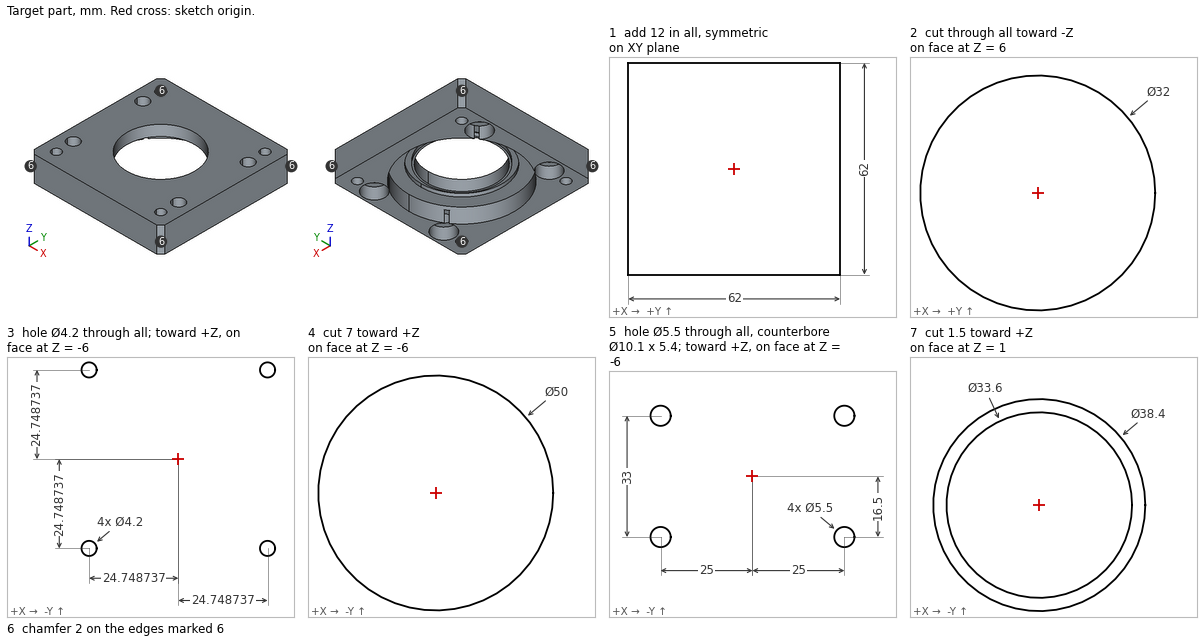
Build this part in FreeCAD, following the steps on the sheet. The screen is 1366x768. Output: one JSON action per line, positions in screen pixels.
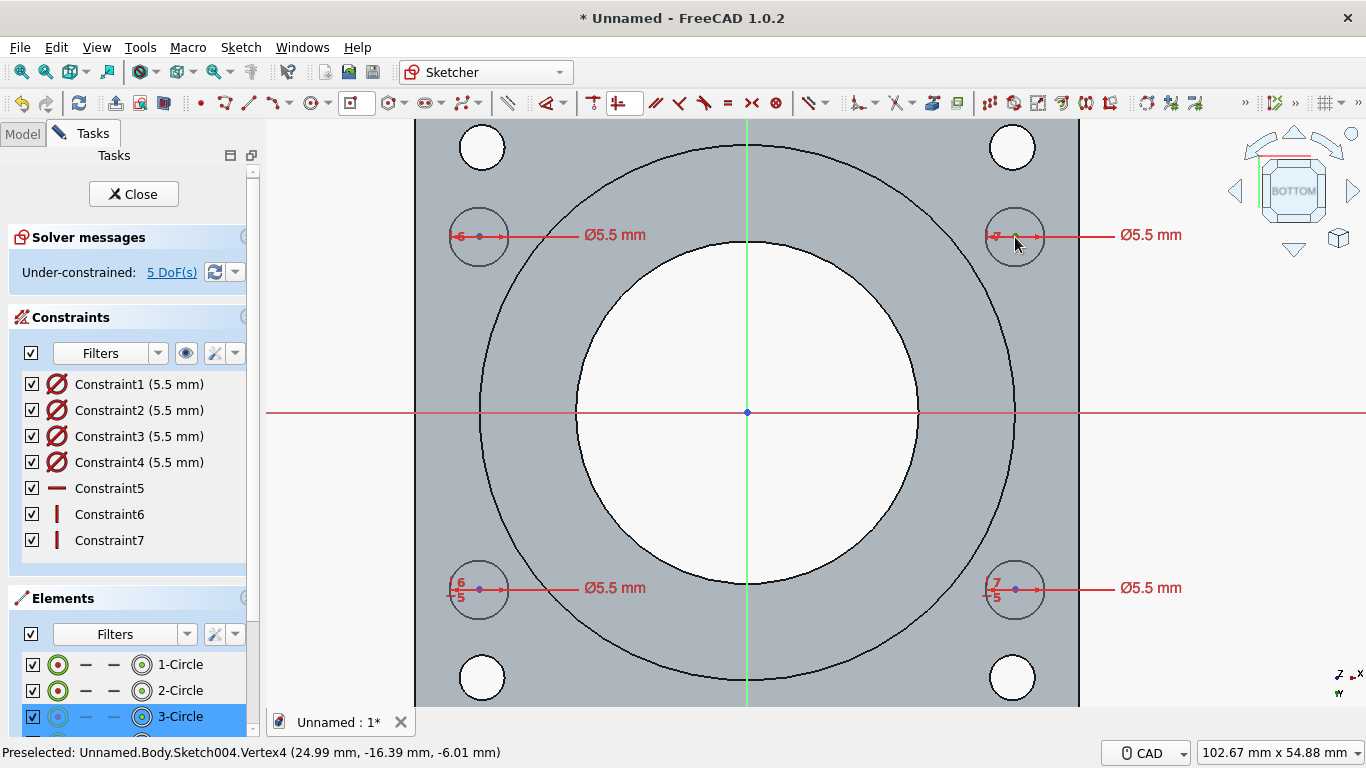
{"action": "left_click", "coordinate": [638, 104]}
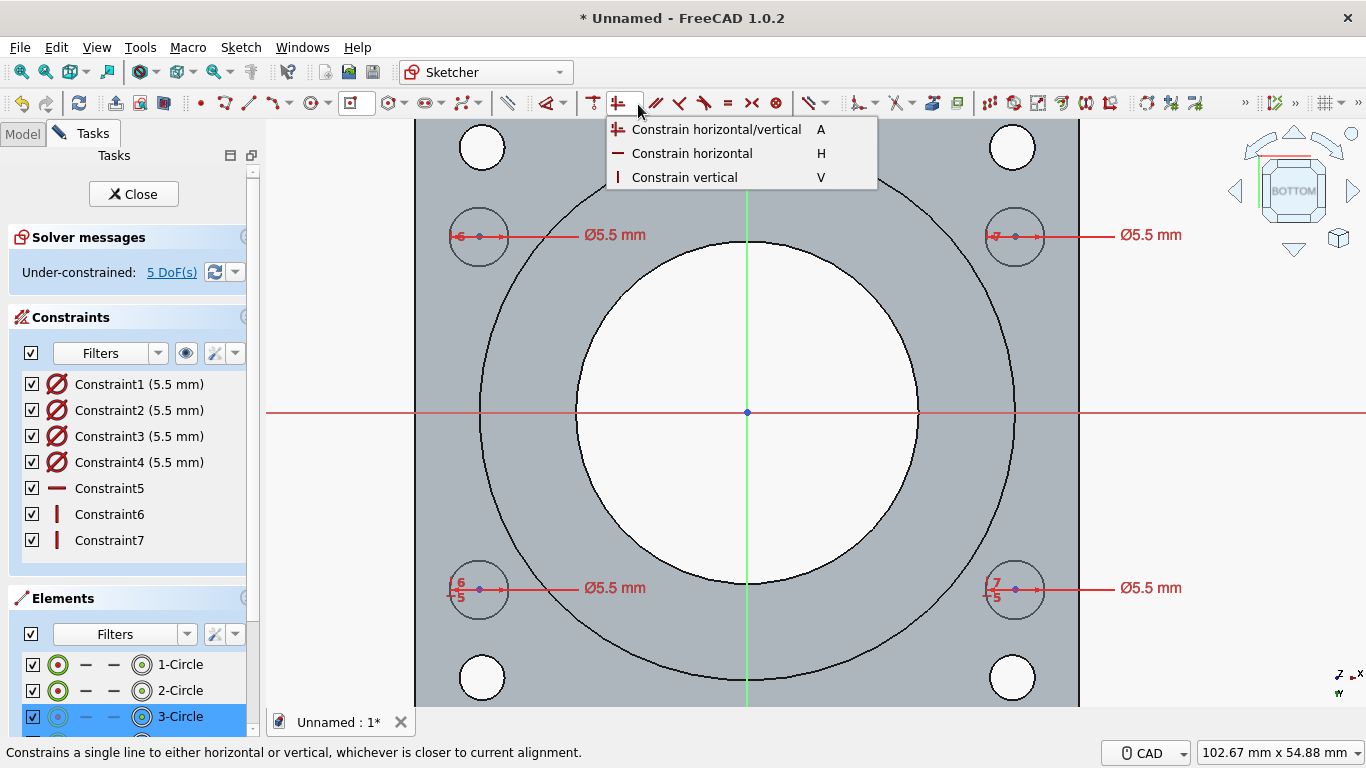
{"action": "left_click", "coordinate": [742, 153]}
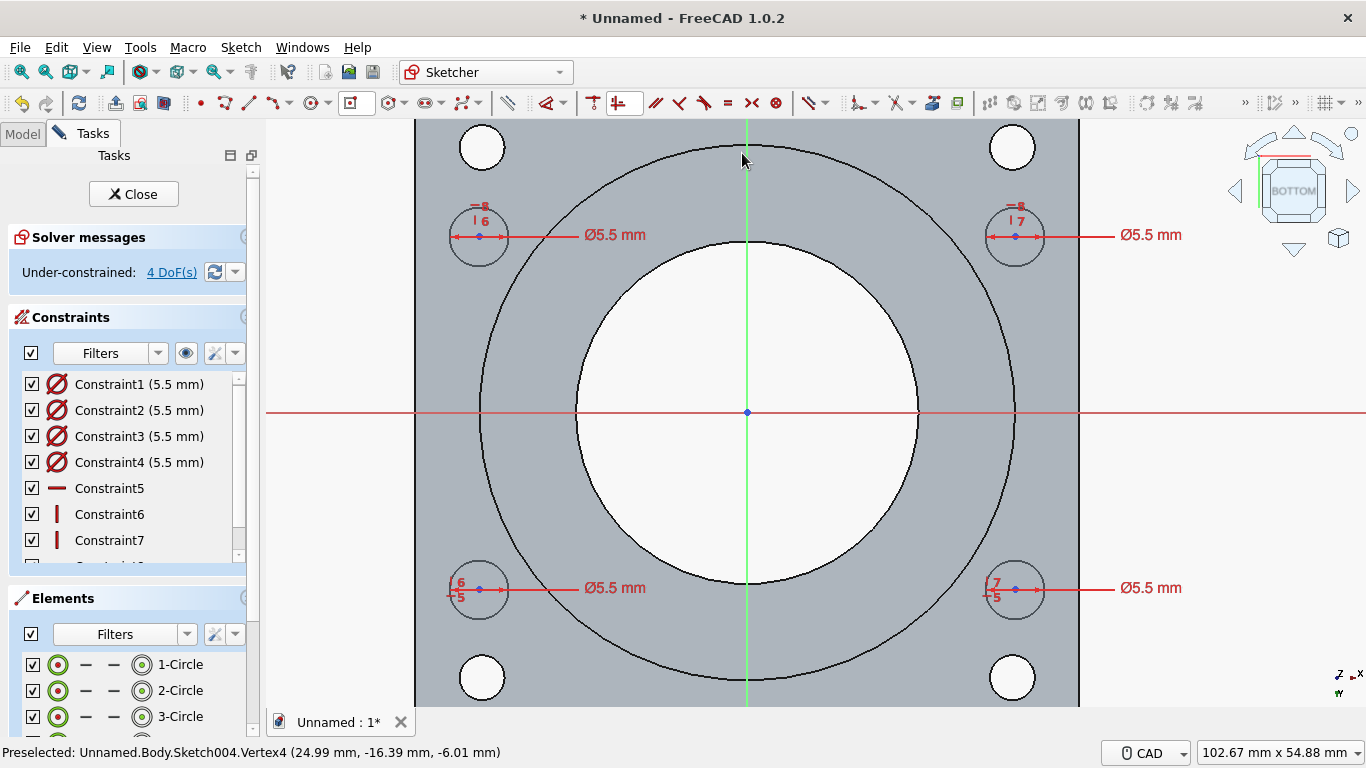
{"action": "left_click", "coordinate": [546, 104]}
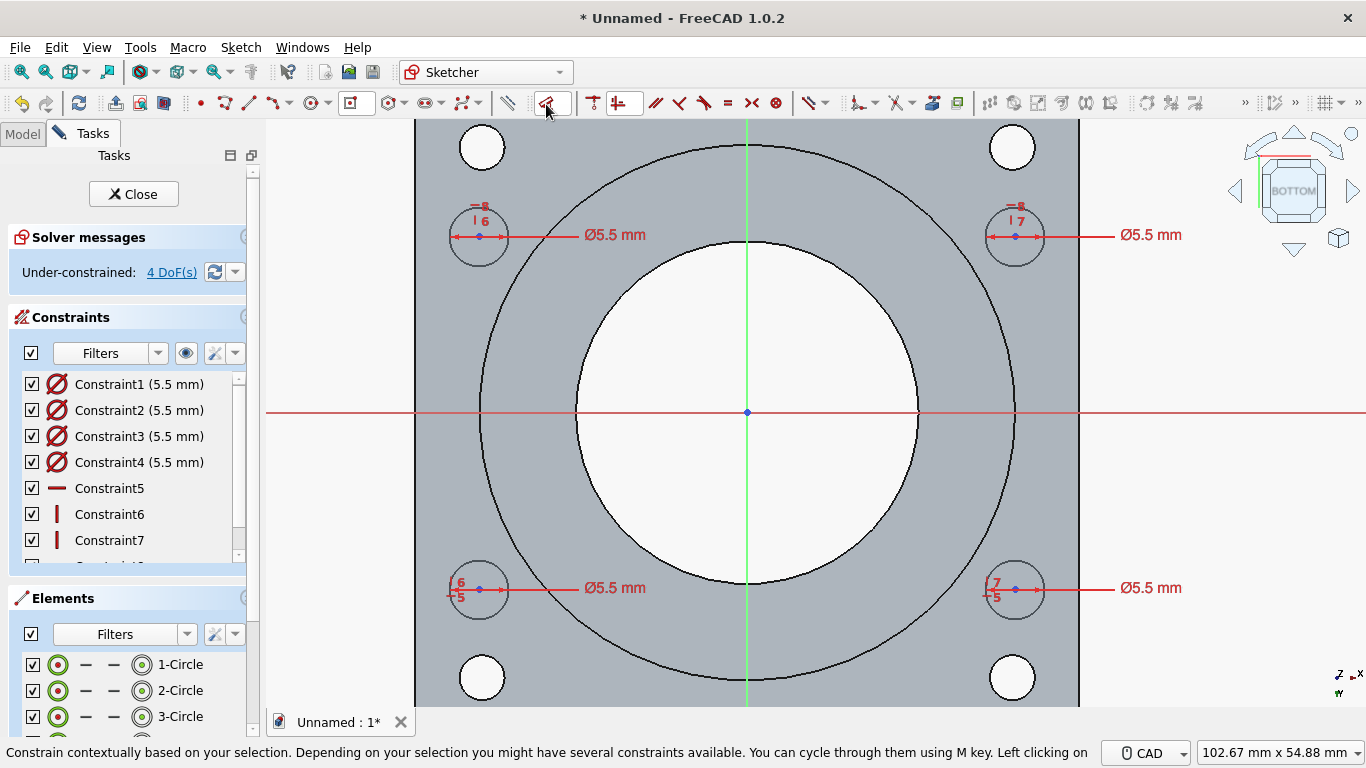
{"action": "left_click", "coordinate": [1015, 590]}
{"action": "left_click", "coordinate": [881, 624]}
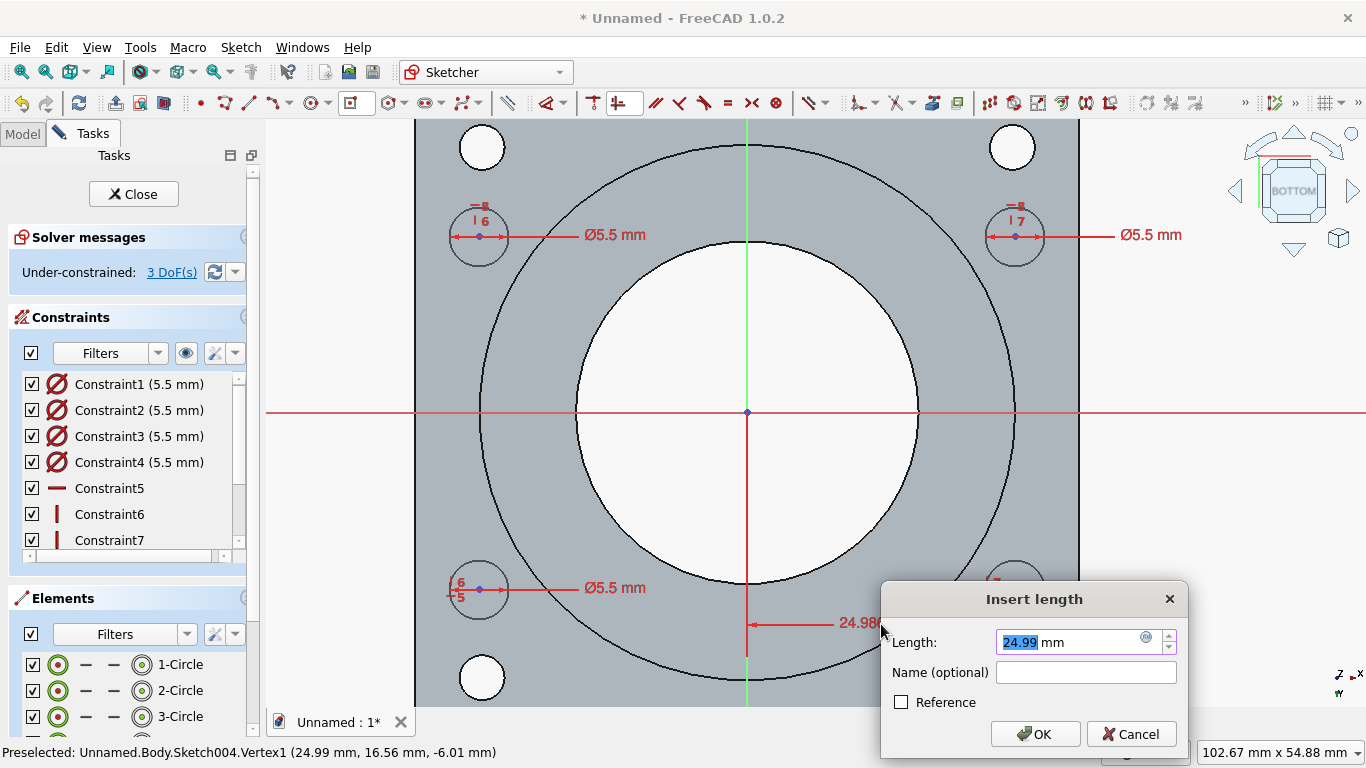
{"action": "type", "text": "25"}
{"action": "key", "text": "Return"}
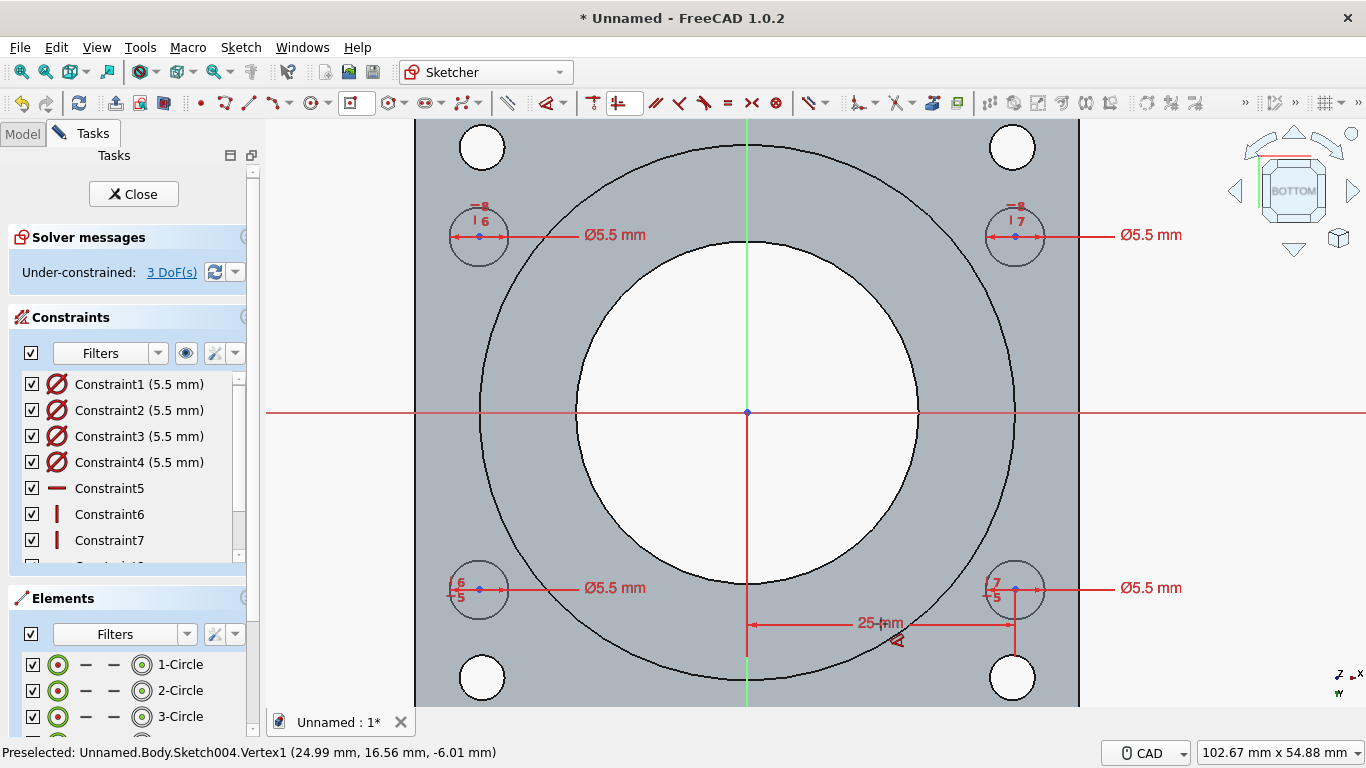
{"action": "left_click", "coordinate": [479, 590]}
{"action": "left_click", "coordinate": [613, 624]}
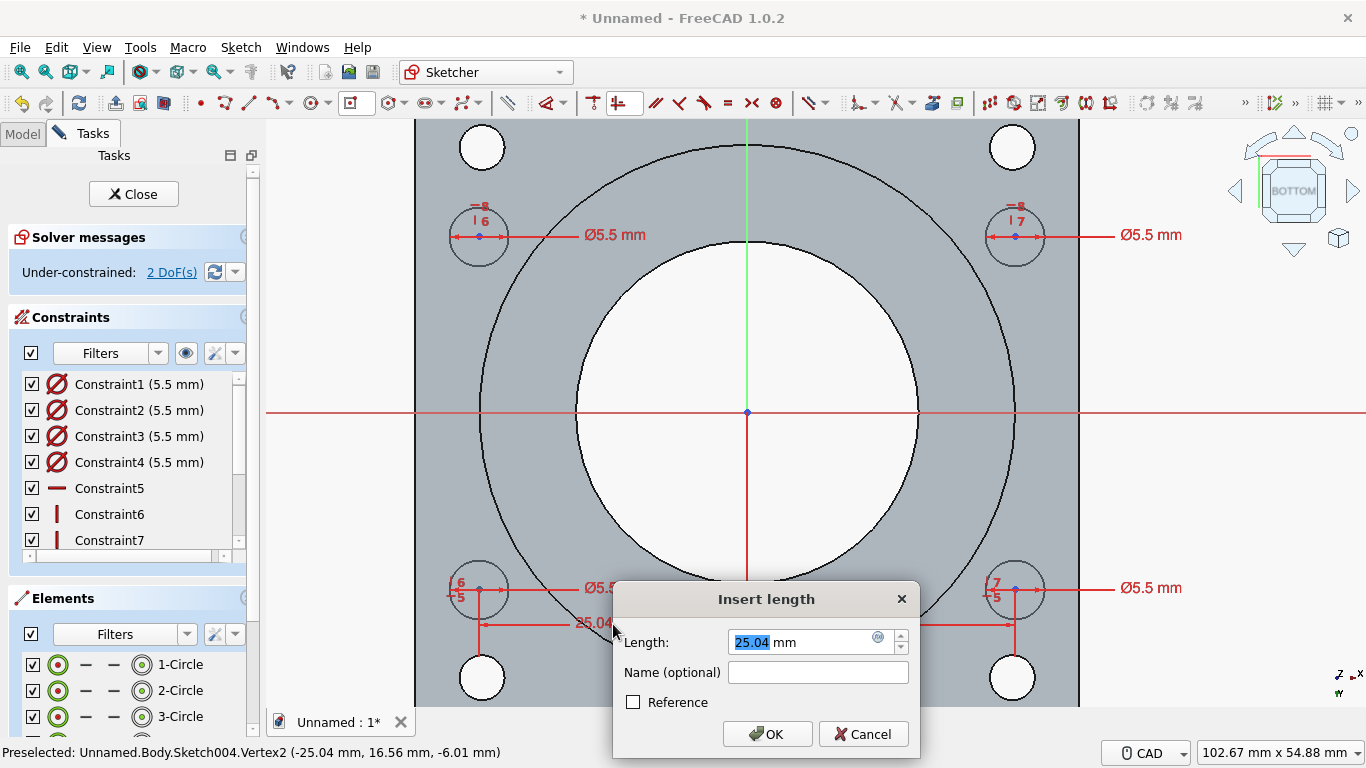
{"action": "type", "text": "25"}
{"action": "key", "text": "Return"}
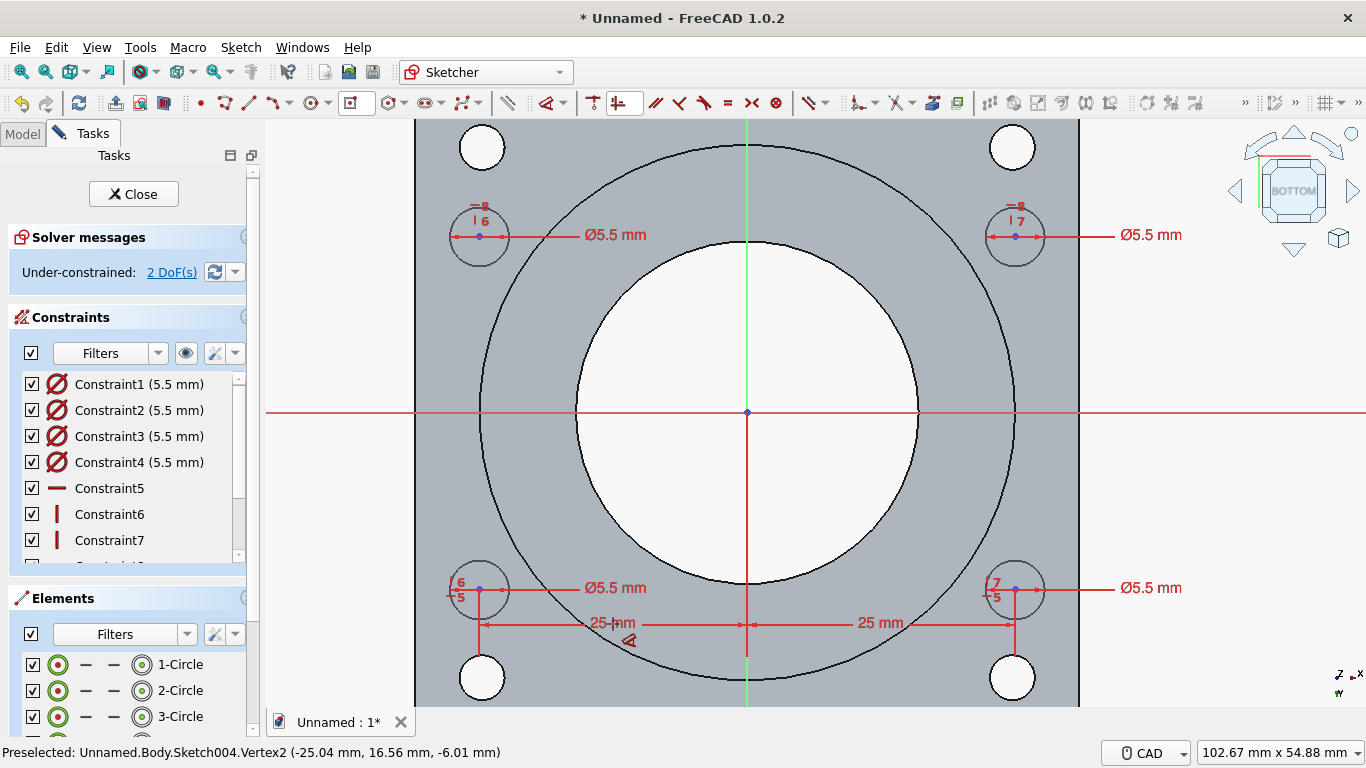
{"action": "left_click", "coordinate": [479, 590]}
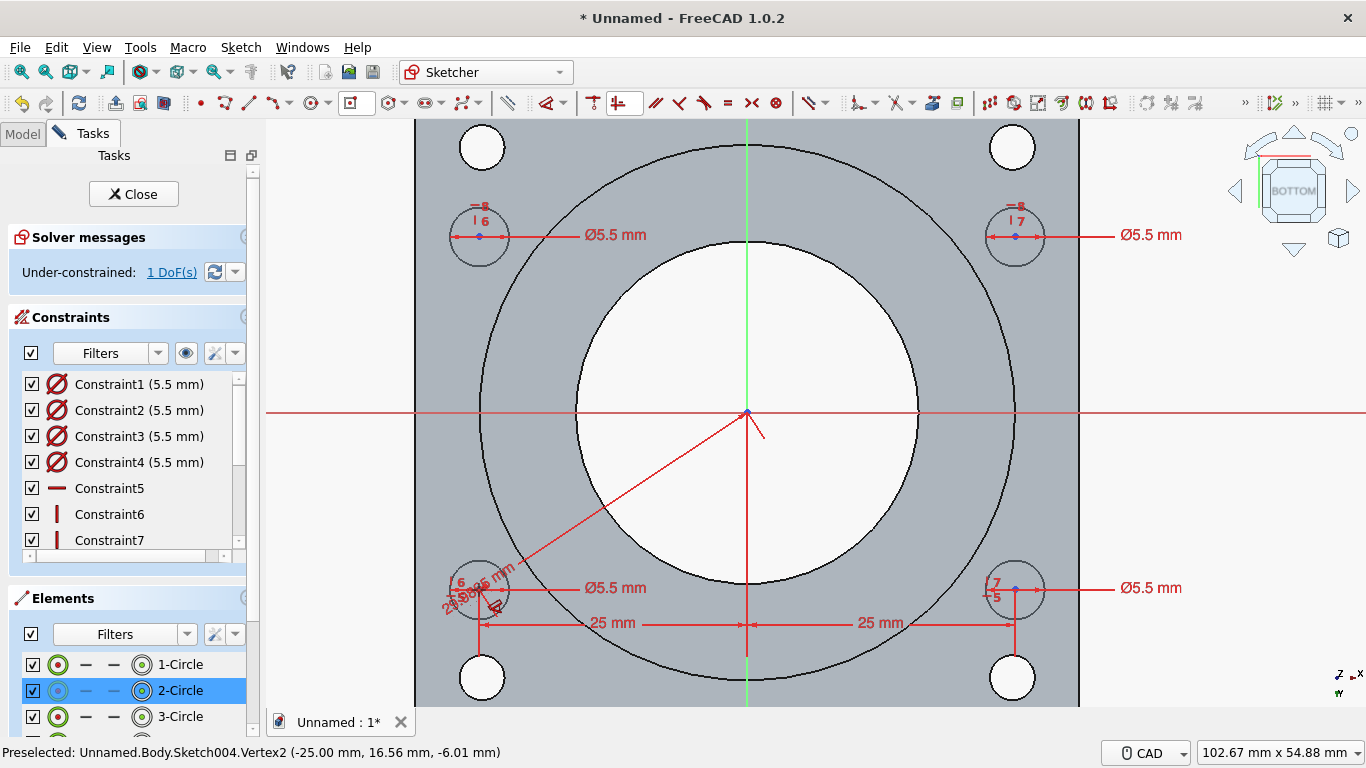
{"action": "left_click", "coordinate": [479, 237]}
{"action": "left_click", "coordinate": [445, 332]}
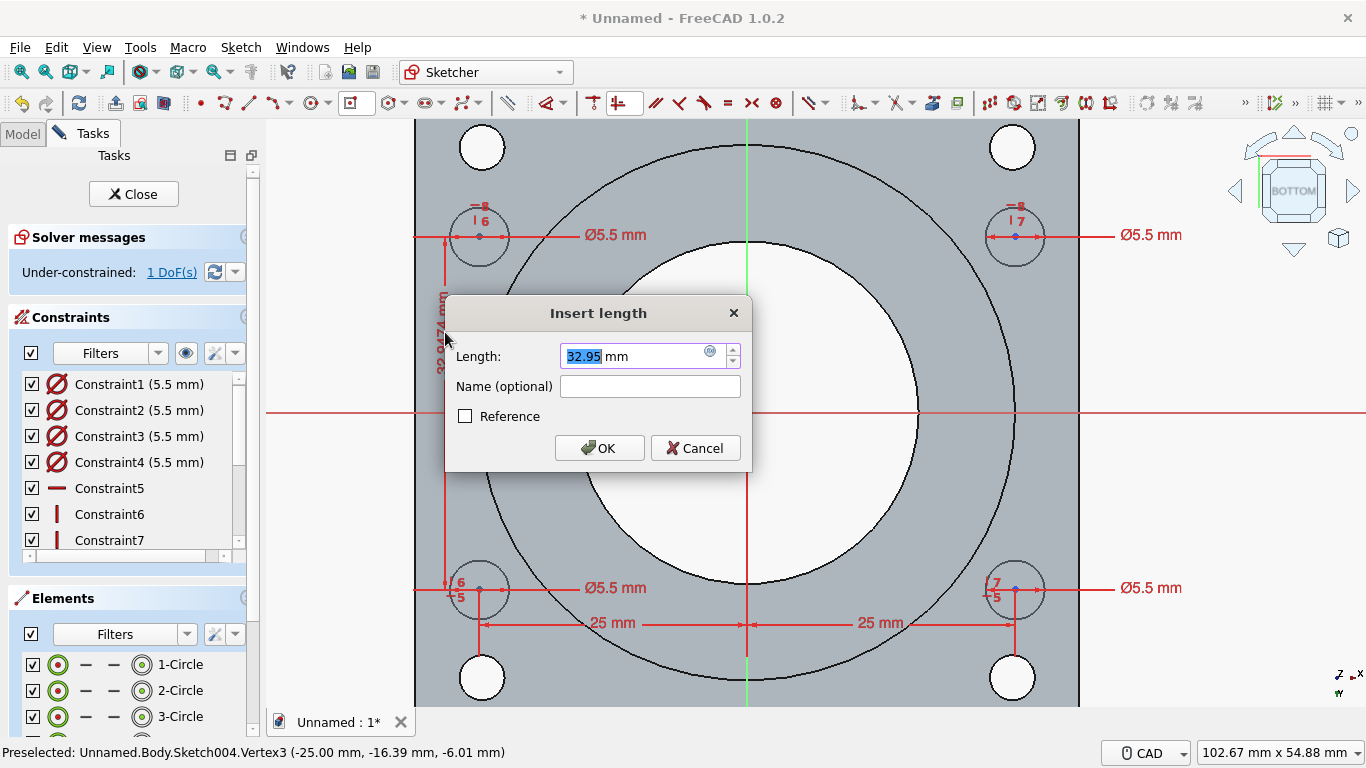
{"action": "type", "text": "33"}
{"action": "key", "text": "Return"}